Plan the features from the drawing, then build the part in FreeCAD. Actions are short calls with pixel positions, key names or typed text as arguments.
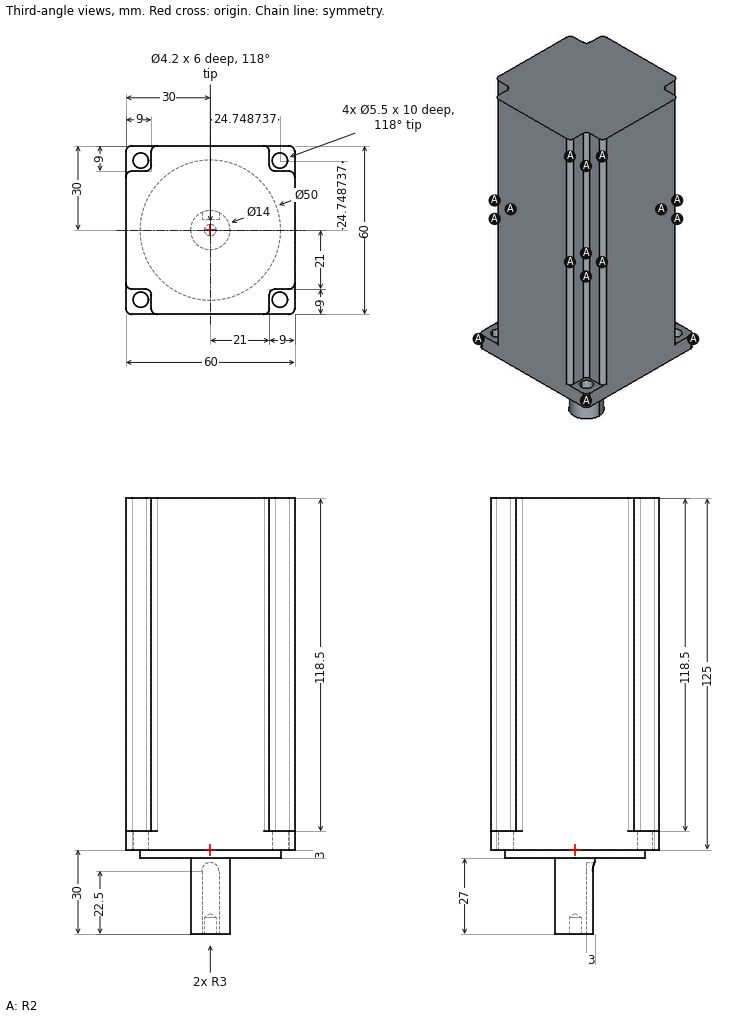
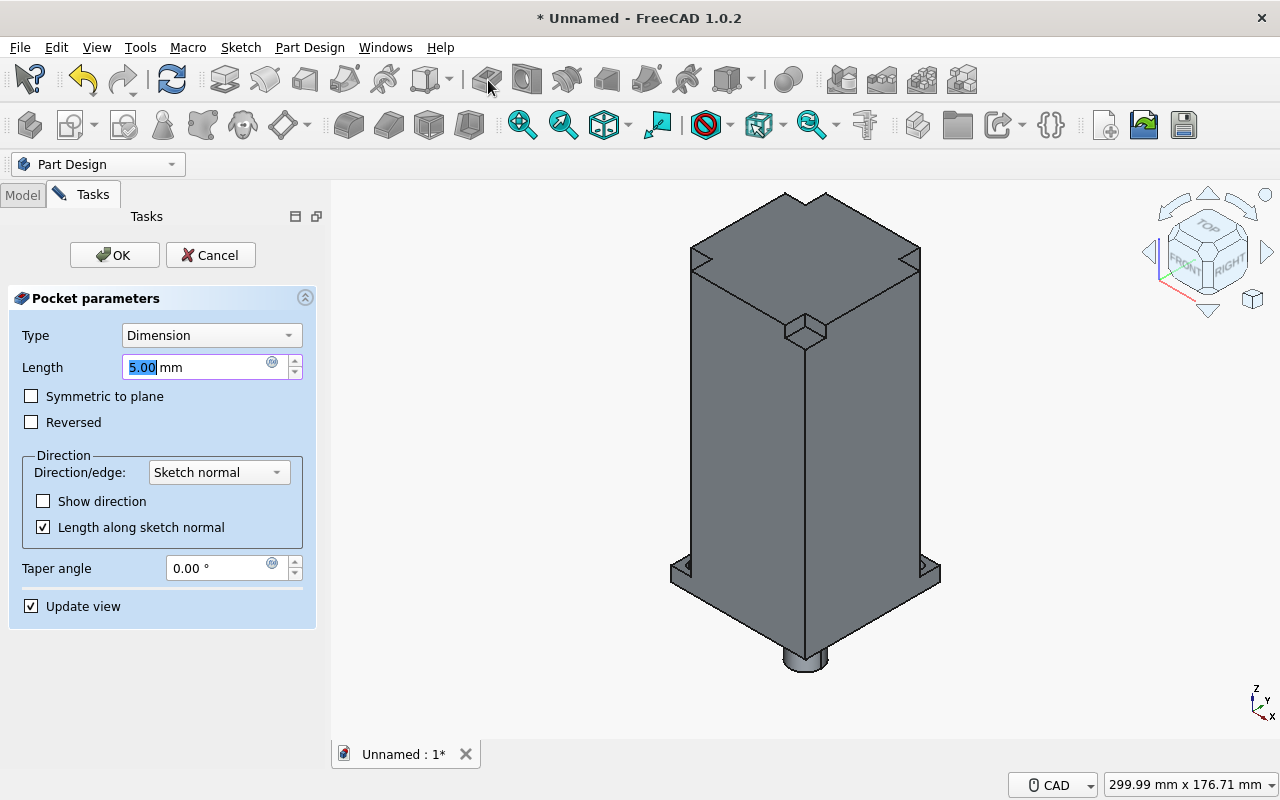
text(118.5)
key(Tab)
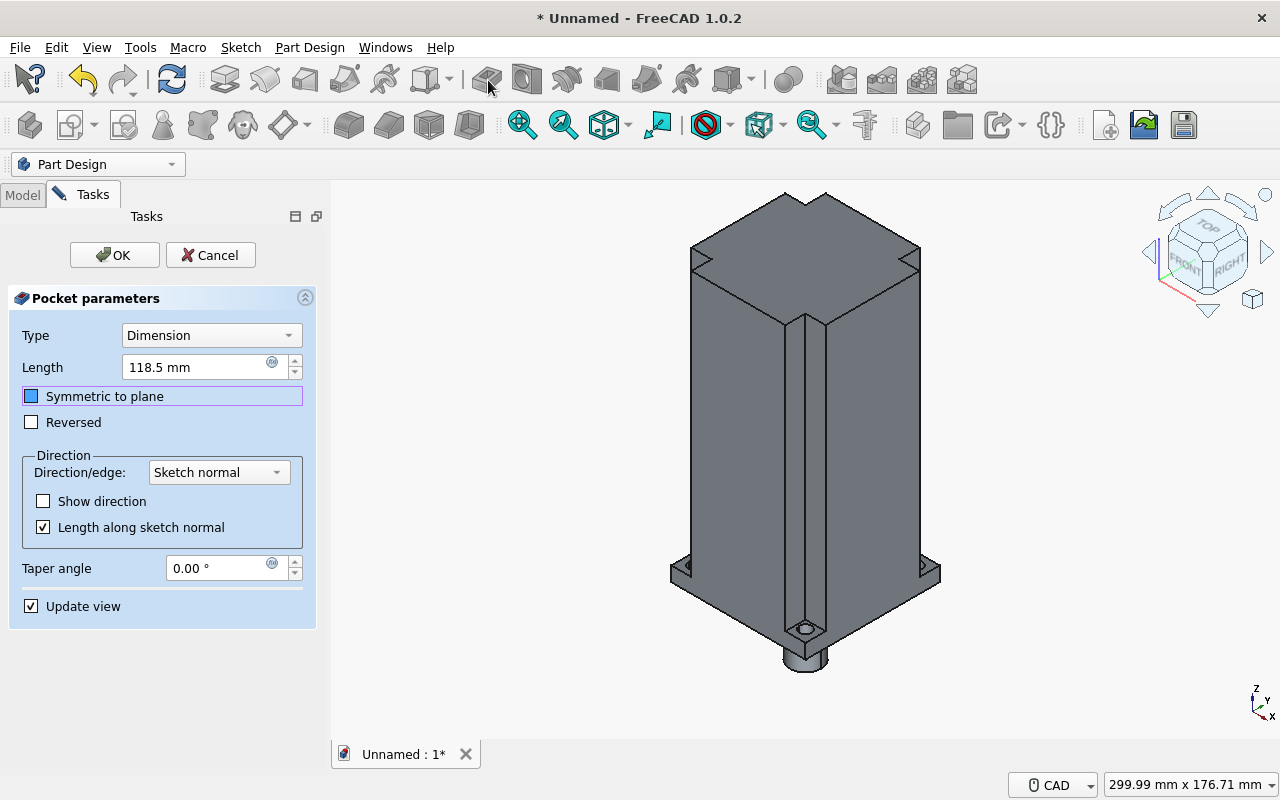
click(115, 255)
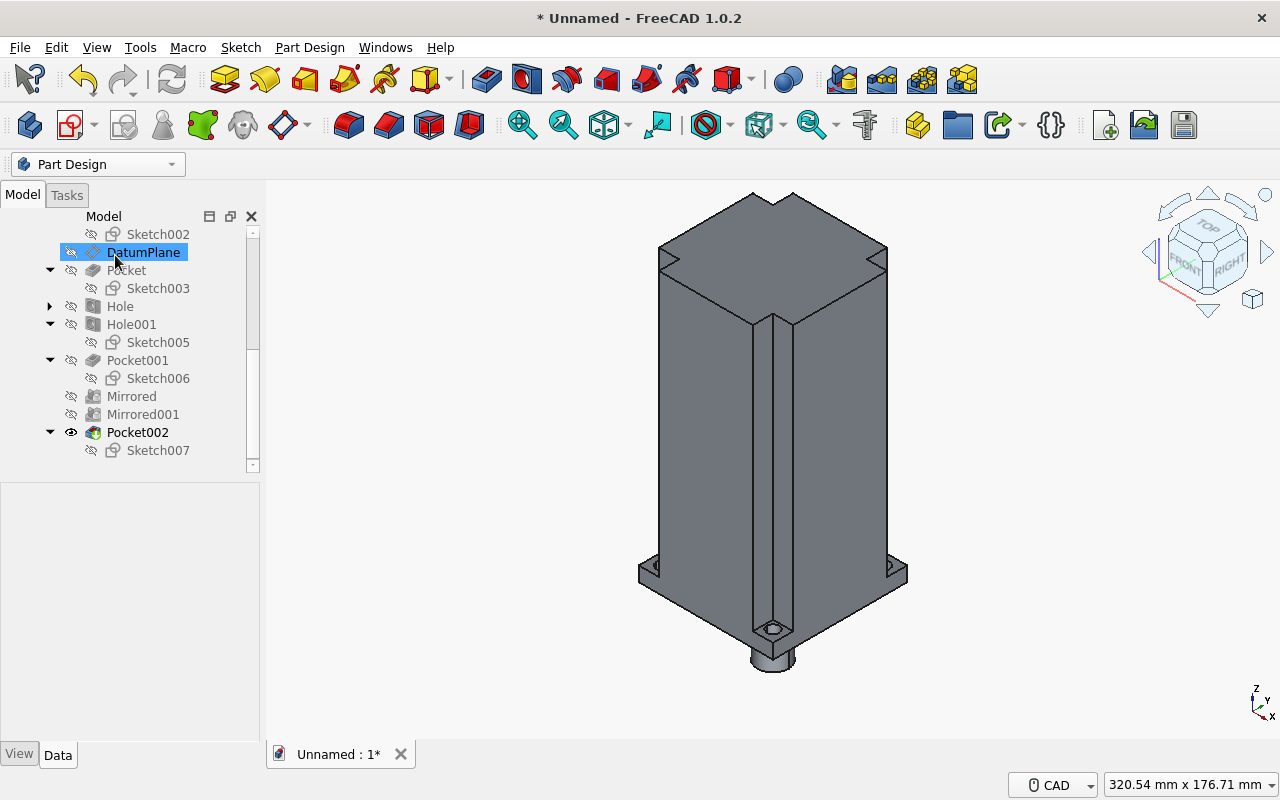
click(773, 650)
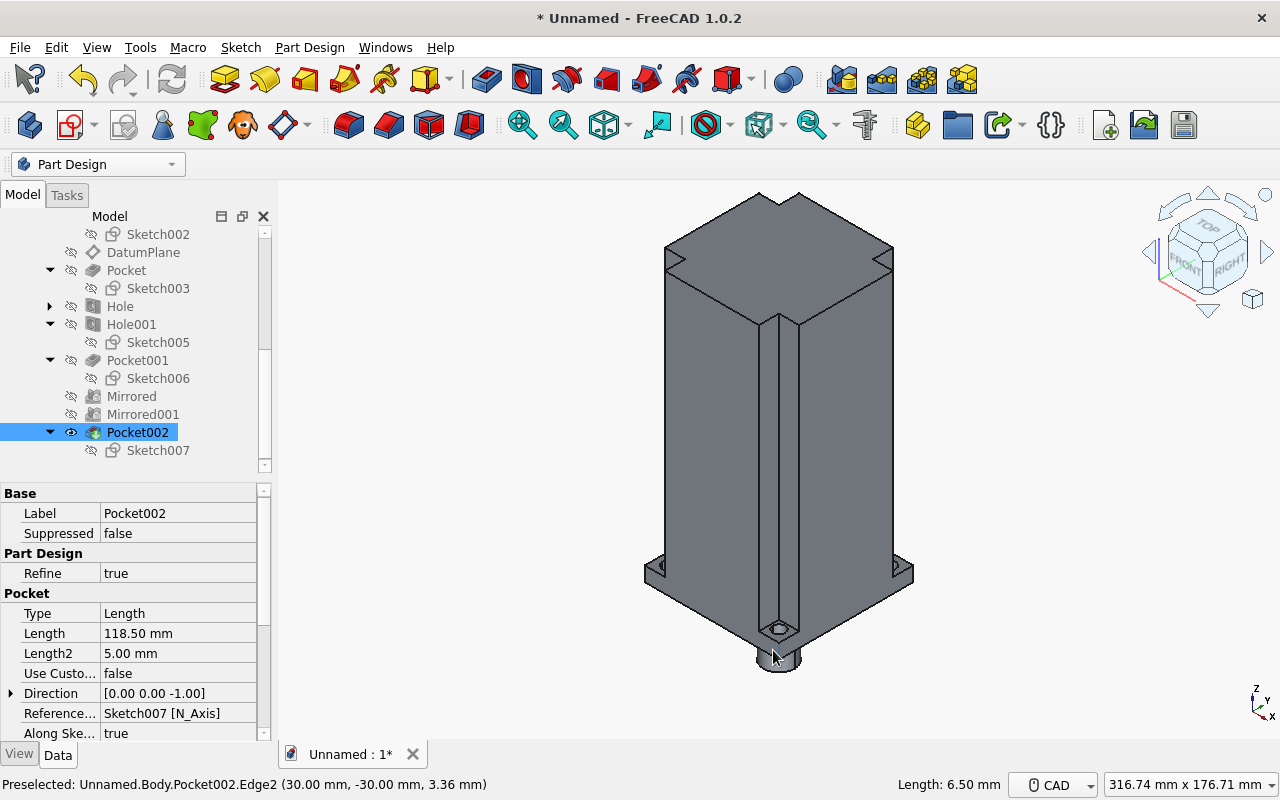
click(799, 477, ctrl)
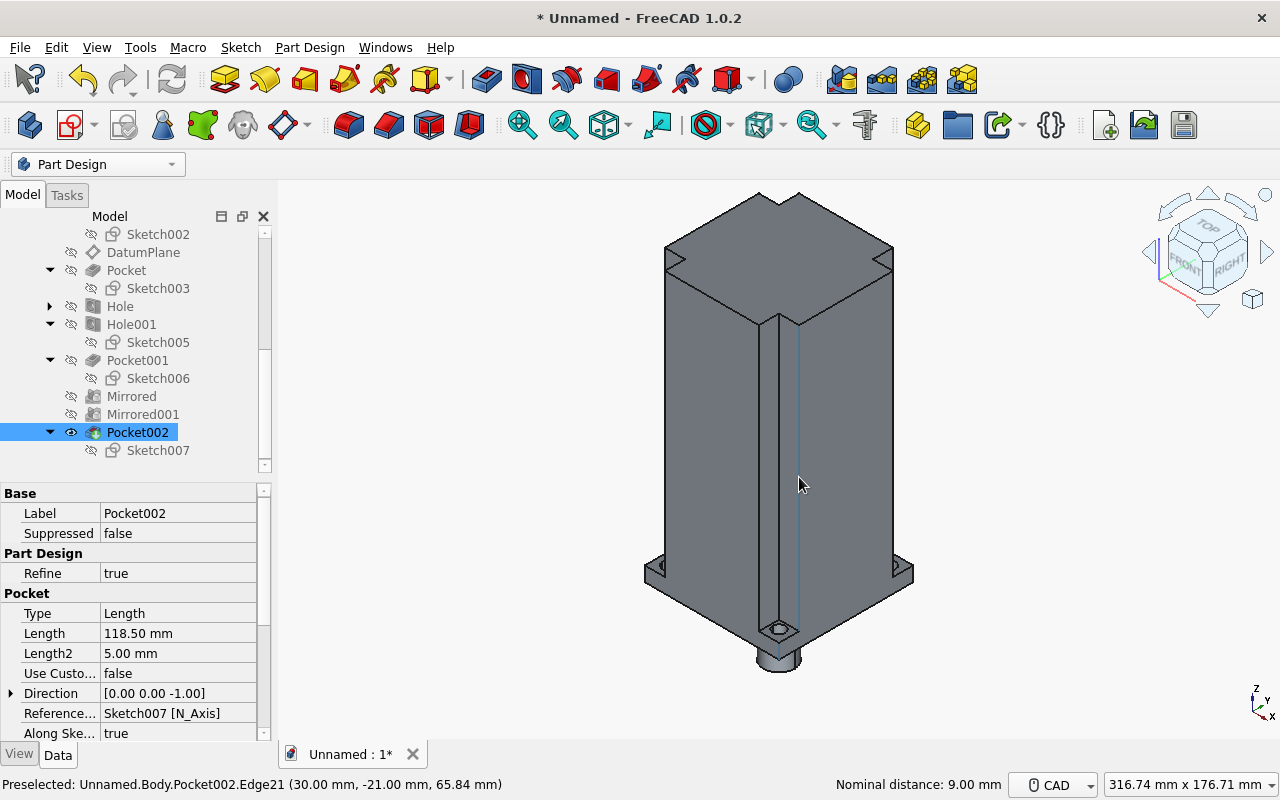
click(759, 477, ctrl)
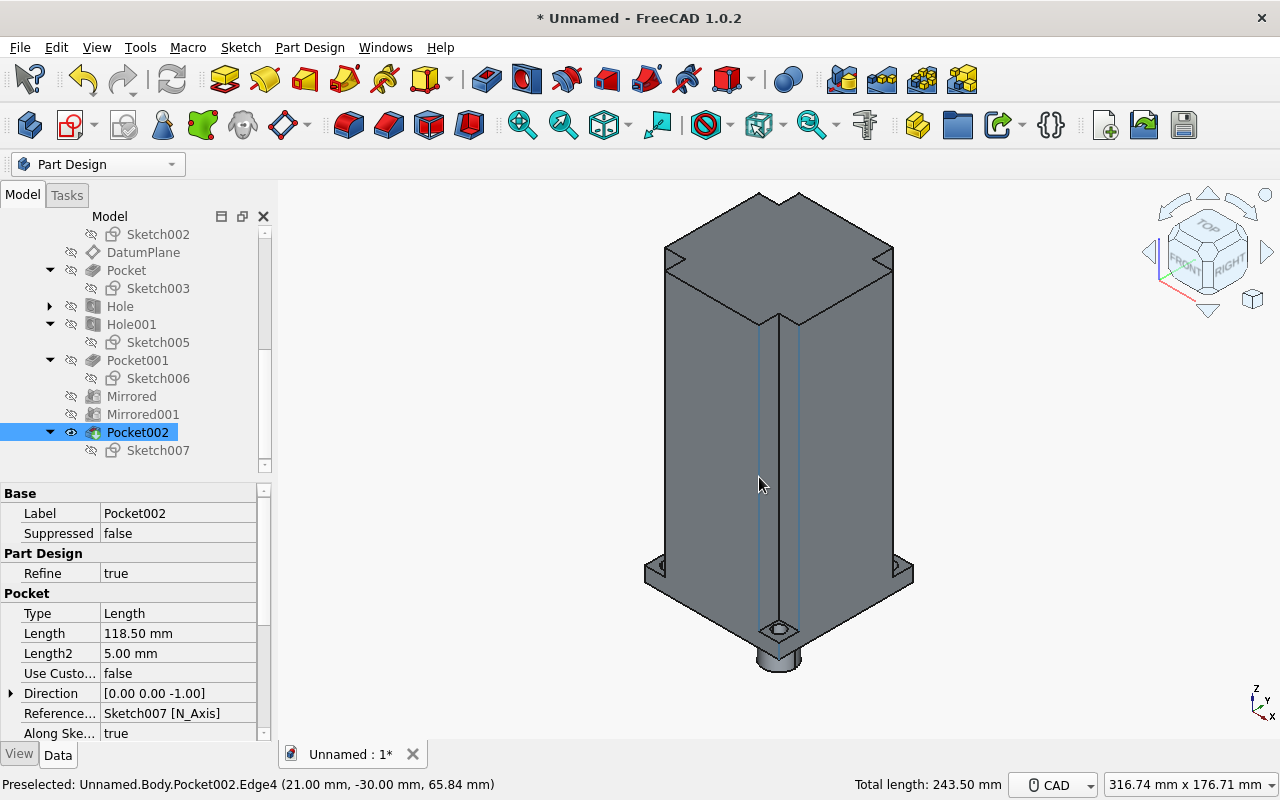
scroll(645, 573, up, 4)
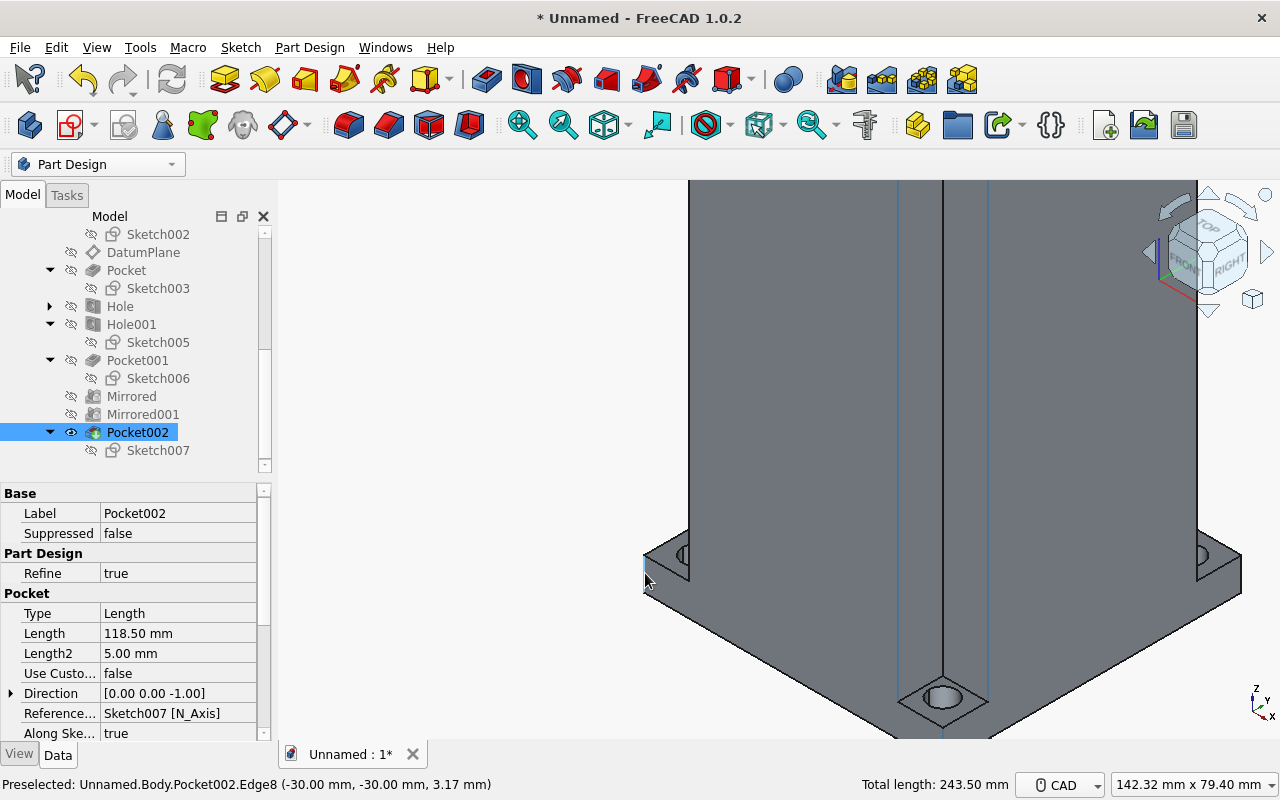
click(524, 126)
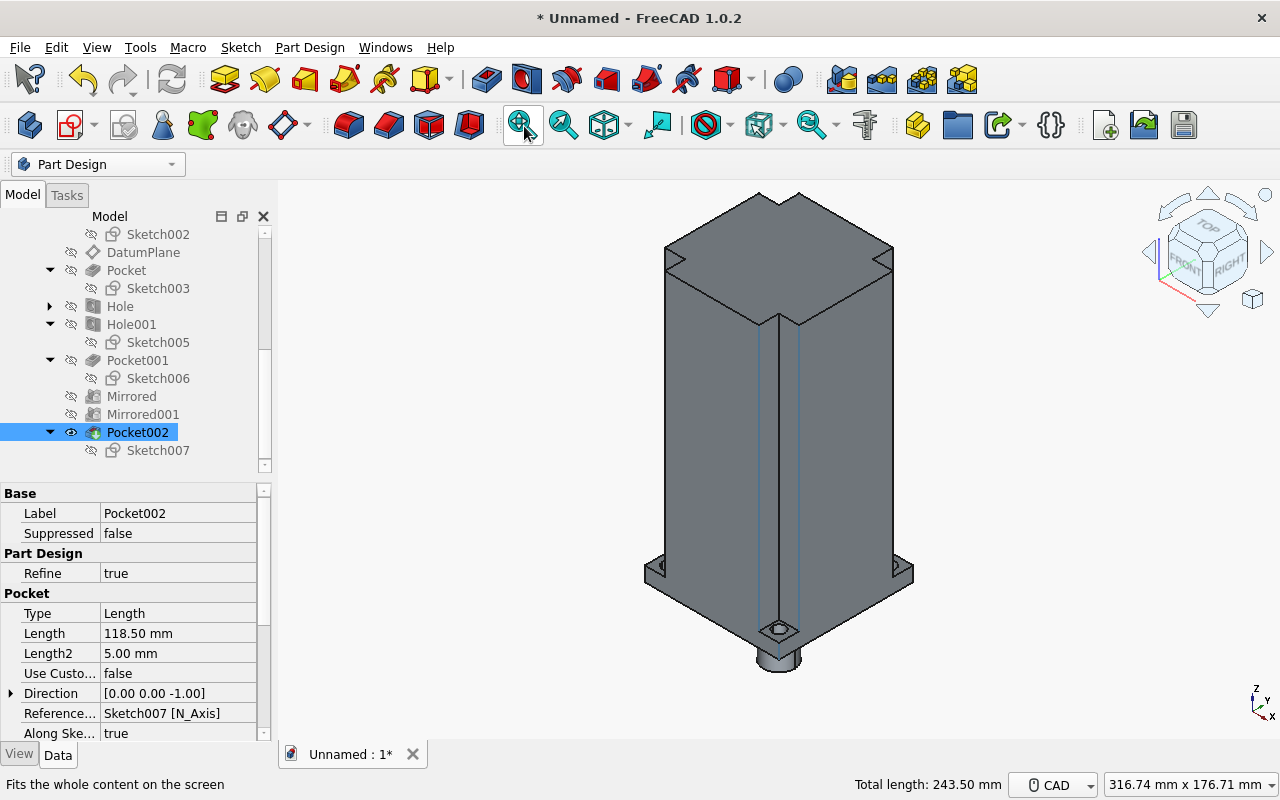
key(2)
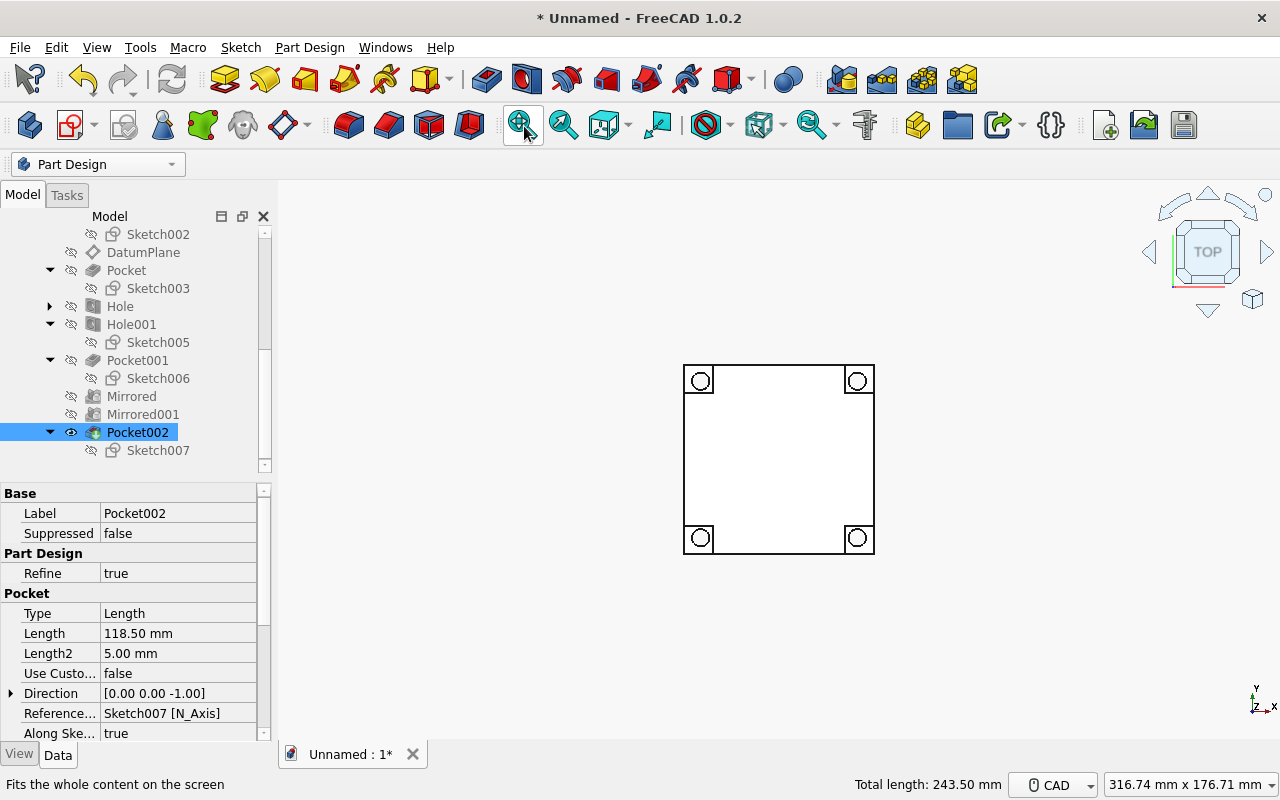
click(524, 126)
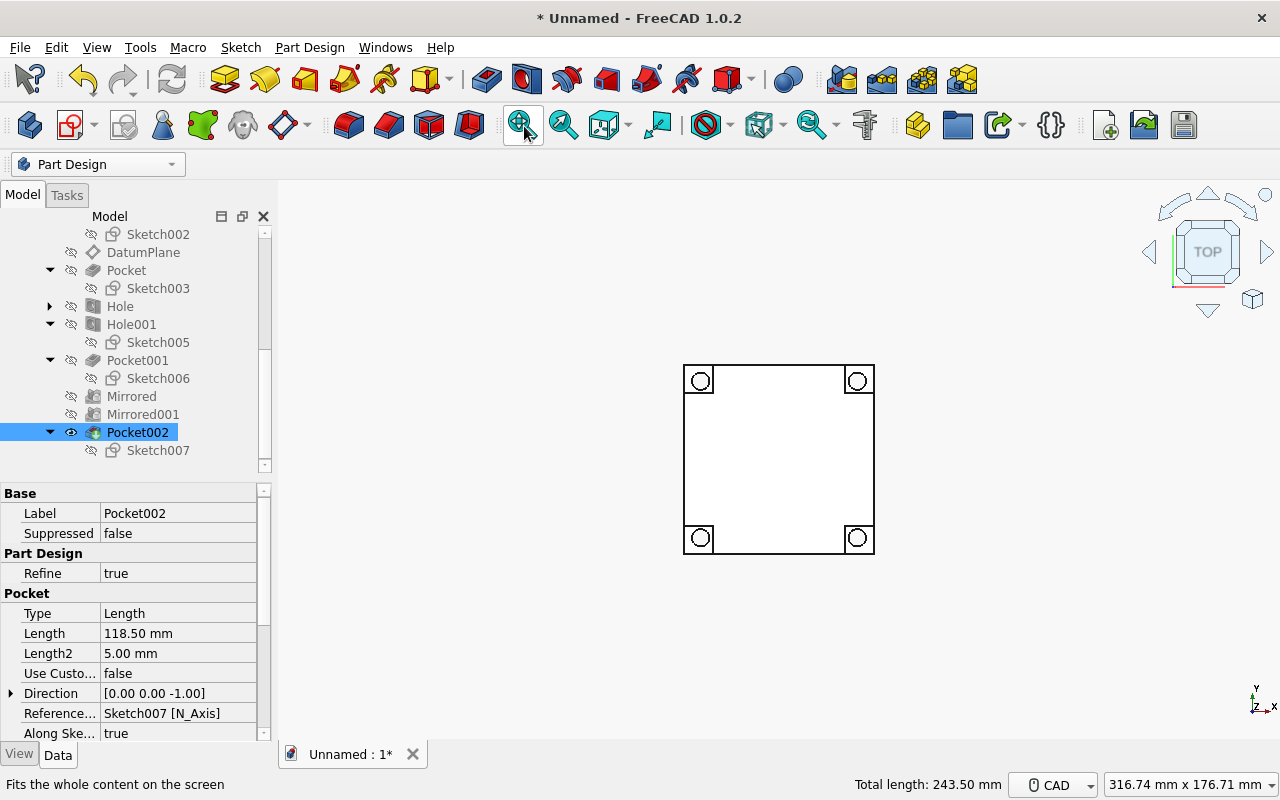
scroll(684, 553, up, 4)